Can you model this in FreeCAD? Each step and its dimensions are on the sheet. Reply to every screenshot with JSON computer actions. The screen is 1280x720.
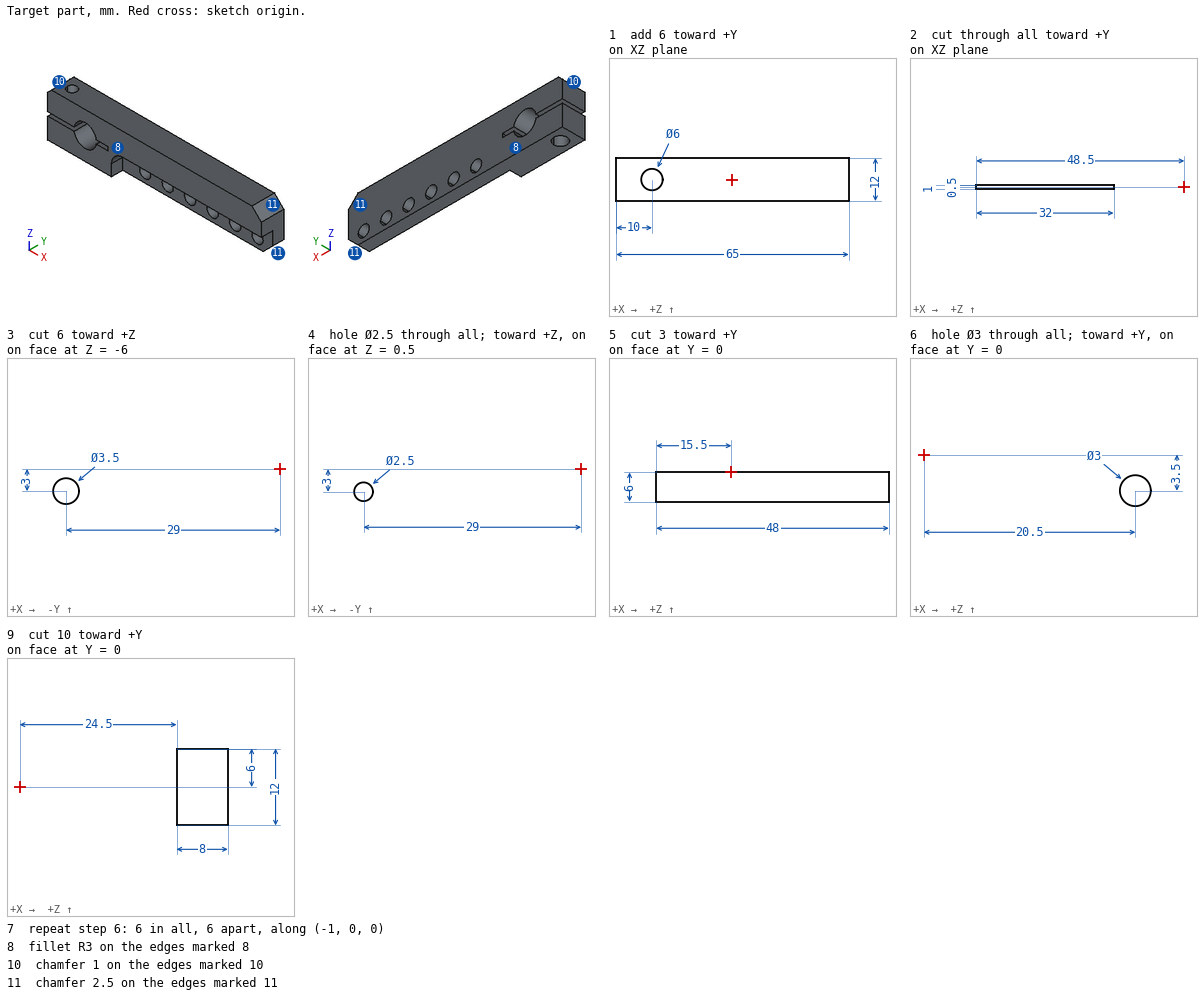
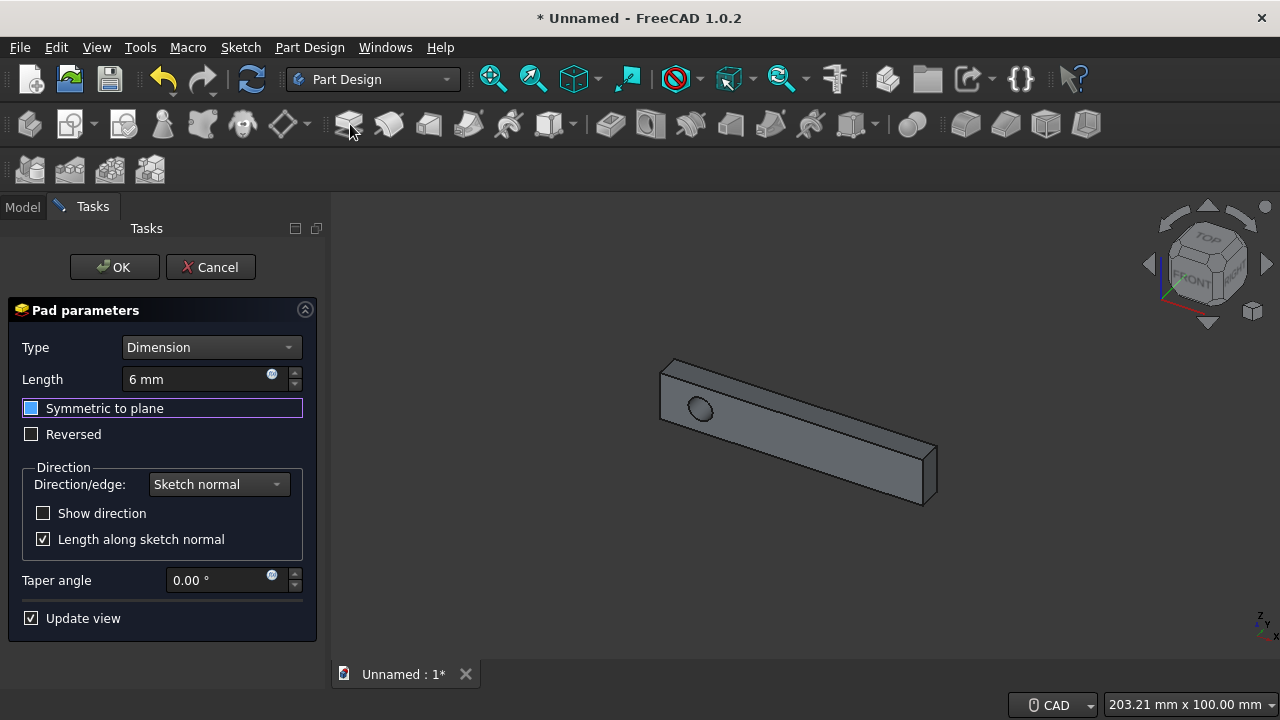
{"action": "left_click", "coordinate": [30, 434]}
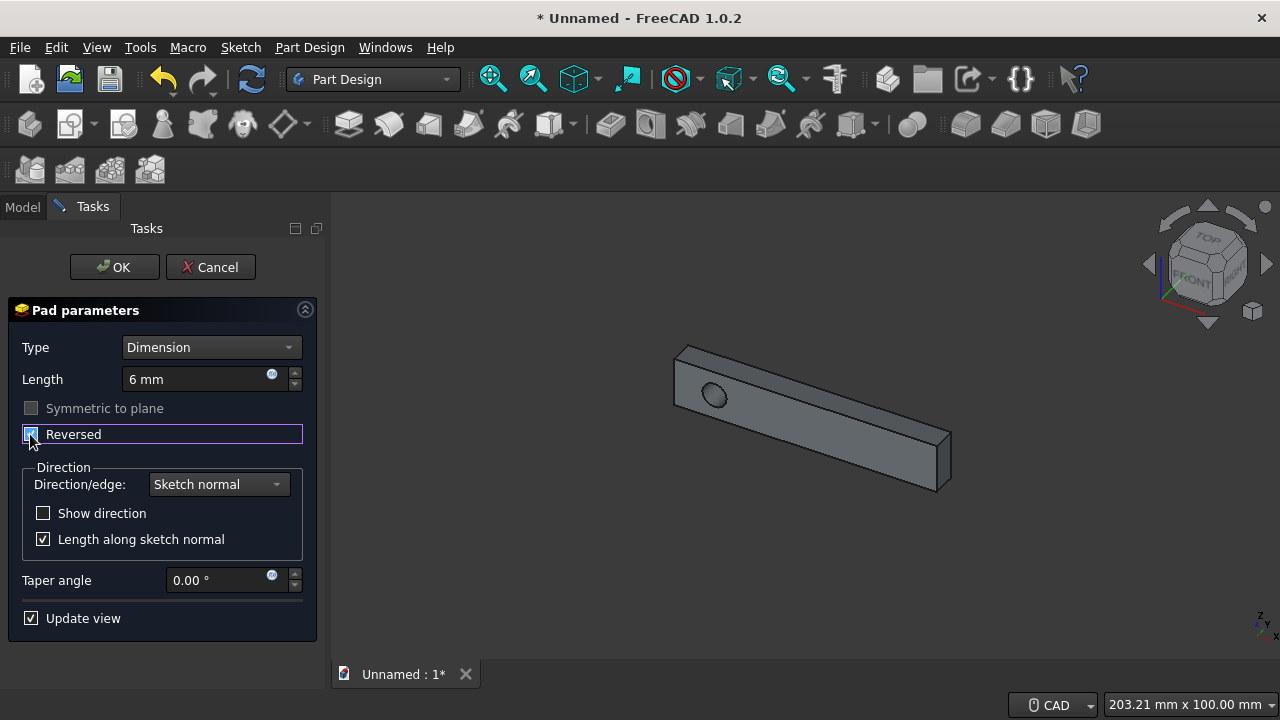
{"action": "left_click", "coordinate": [115, 267]}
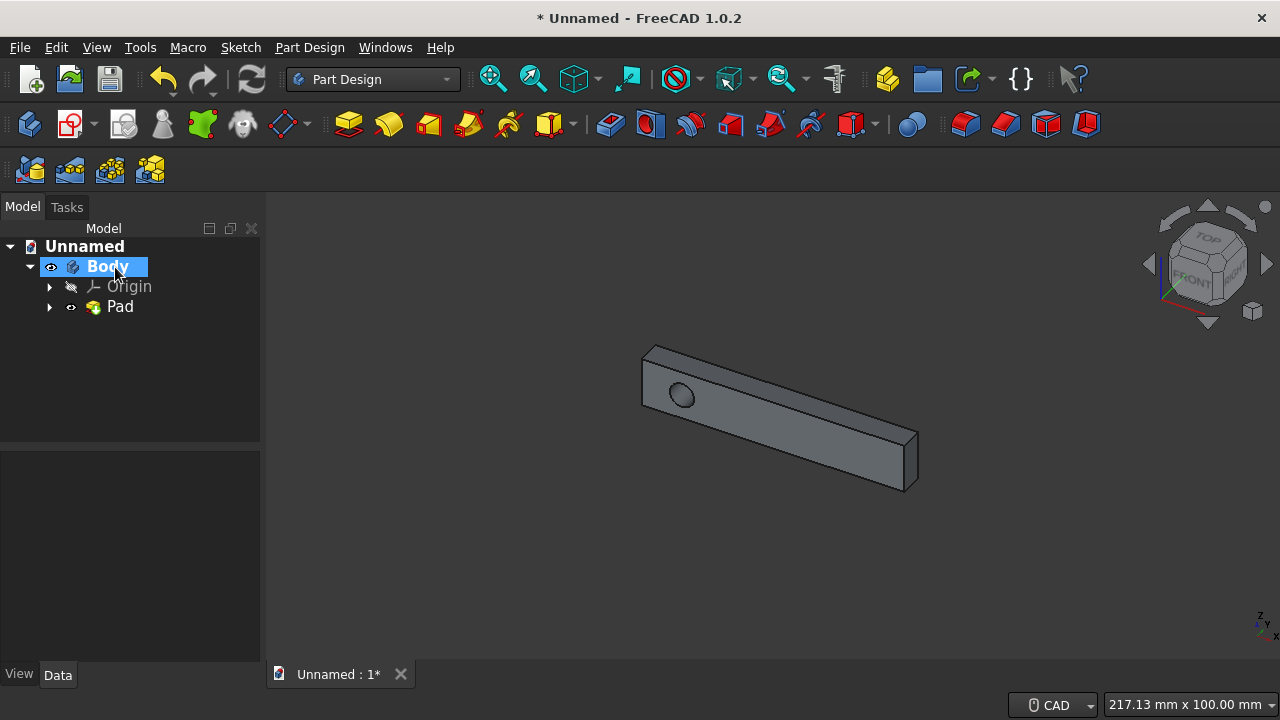
{"action": "left_click", "coordinate": [494, 80]}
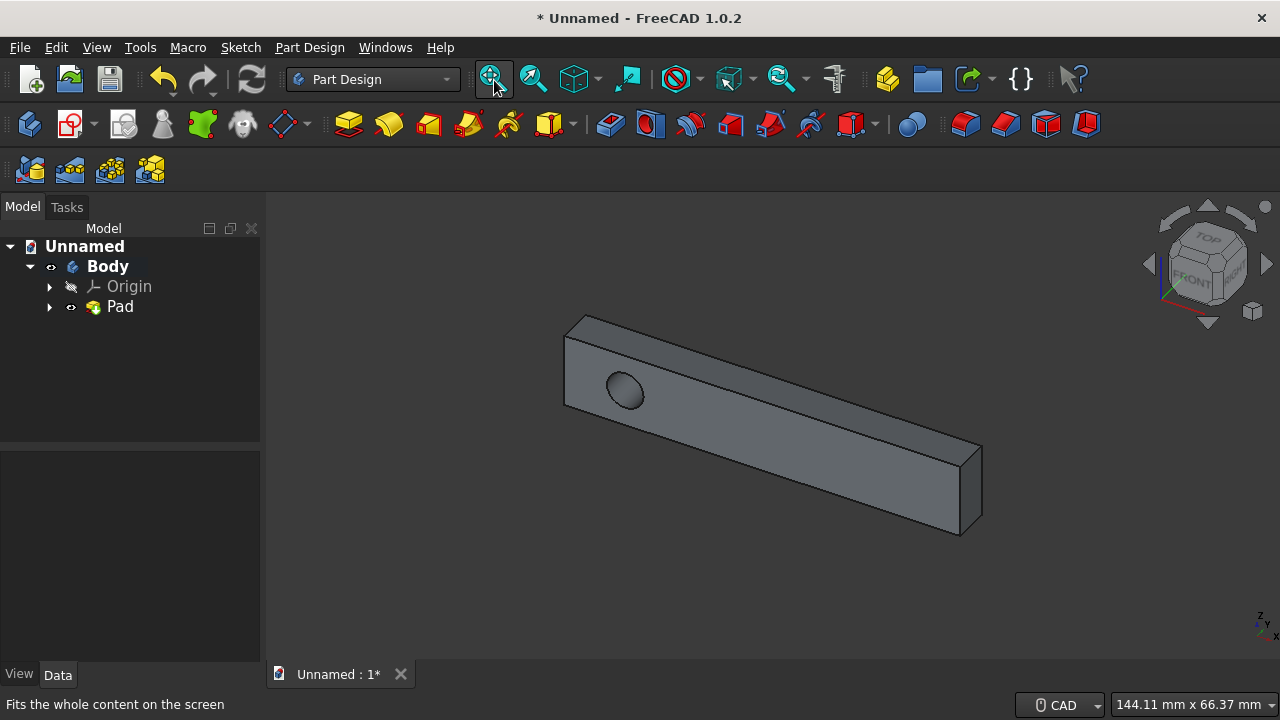
{"action": "left_click", "coordinate": [70, 124]}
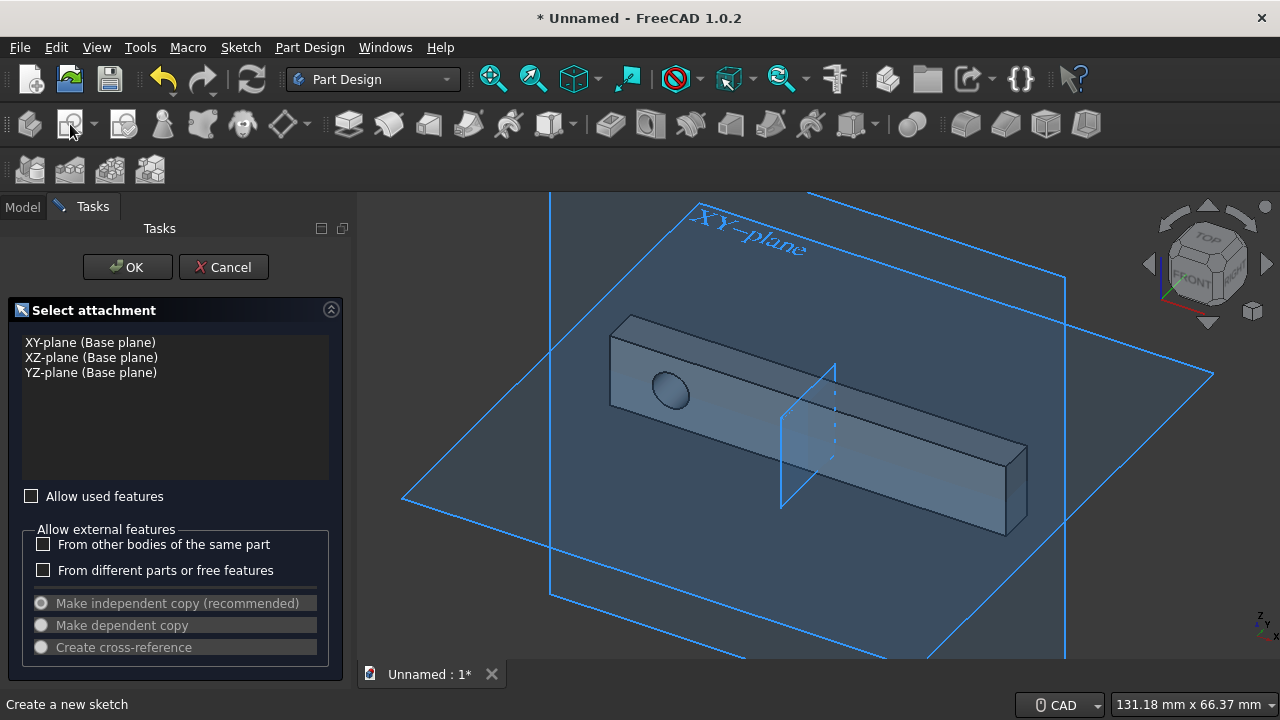
{"action": "left_click", "coordinate": [82, 358]}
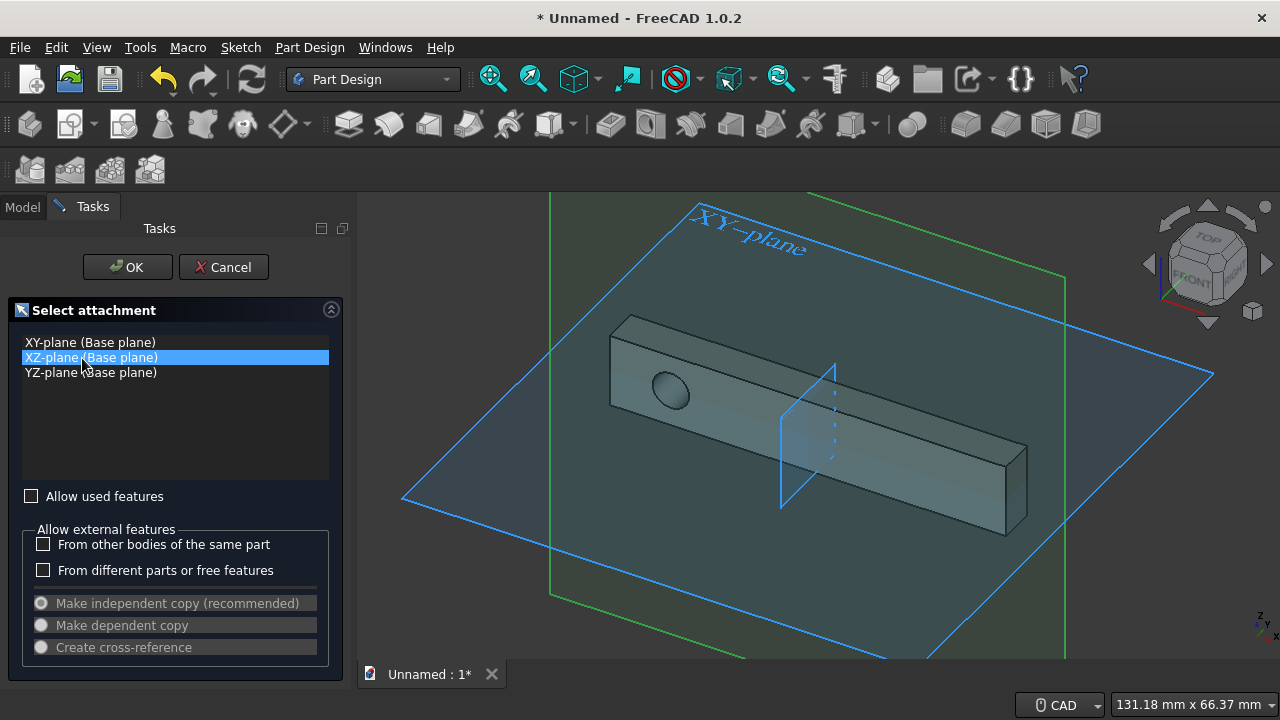
{"action": "left_click", "coordinate": [128, 267]}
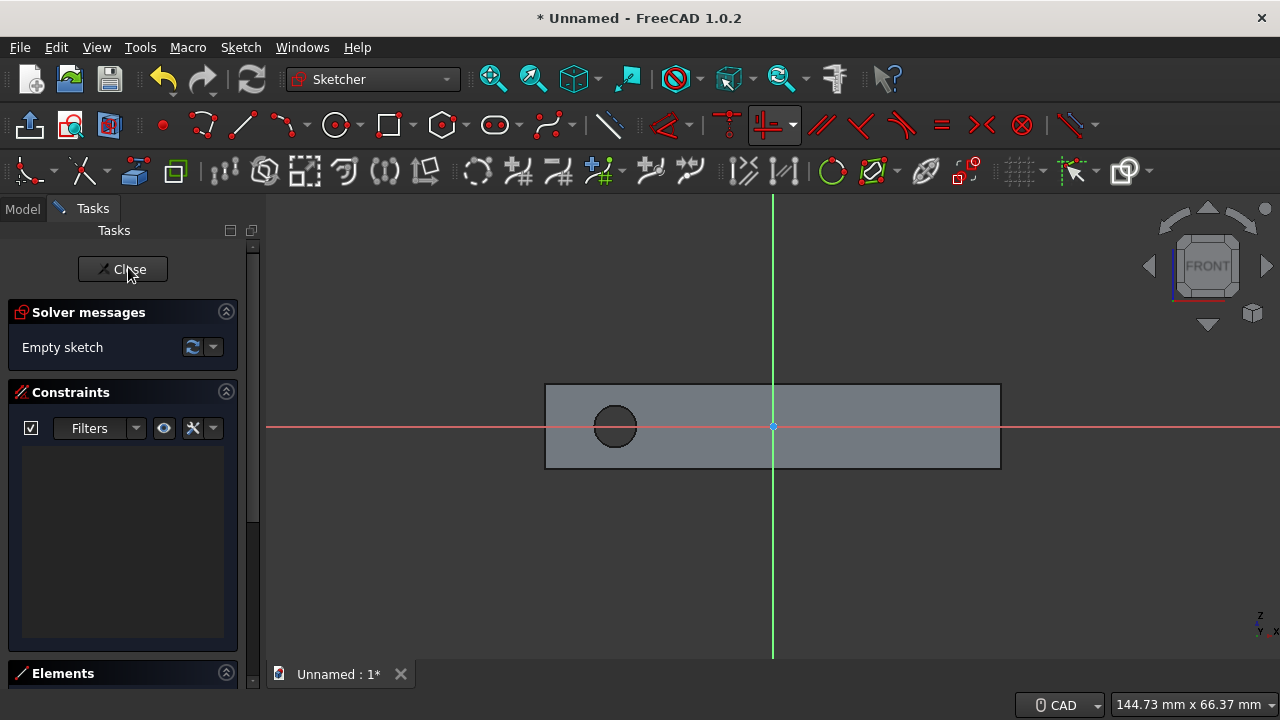
{"action": "scroll", "coordinate": [480, 426], "scroll_direction": "up", "scroll_amount": 3}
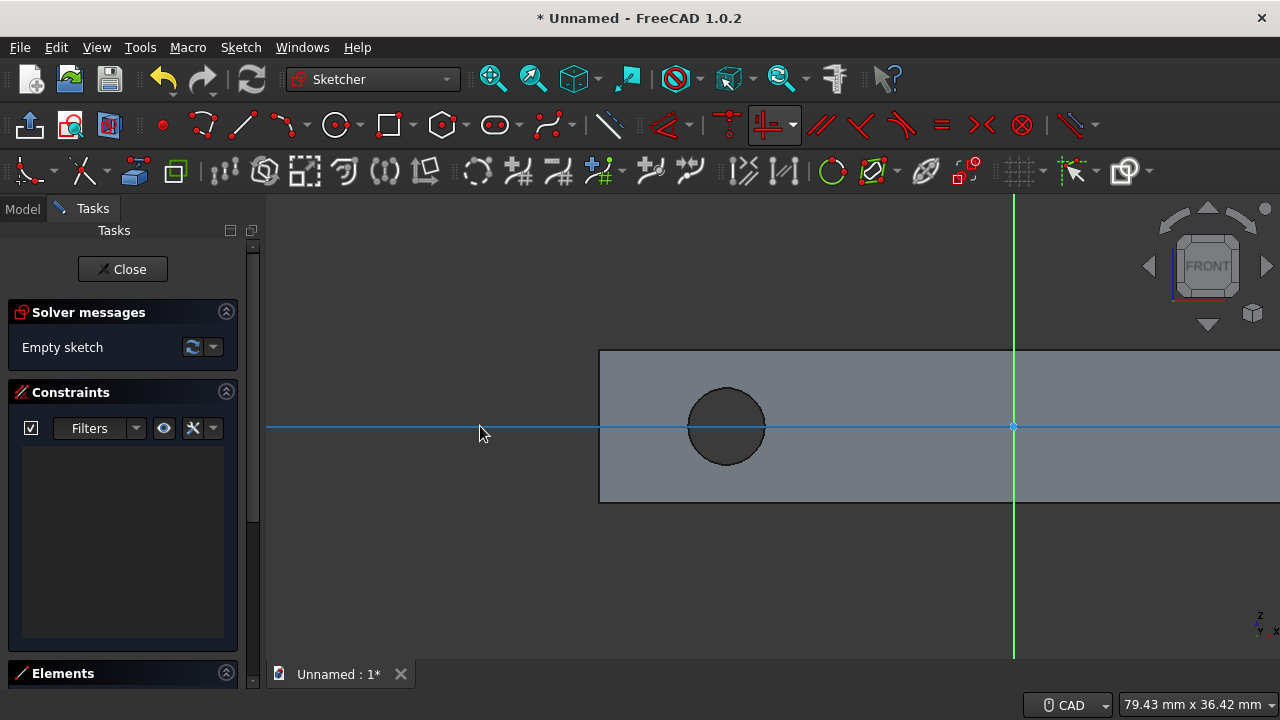
{"action": "left_click", "coordinate": [390, 126]}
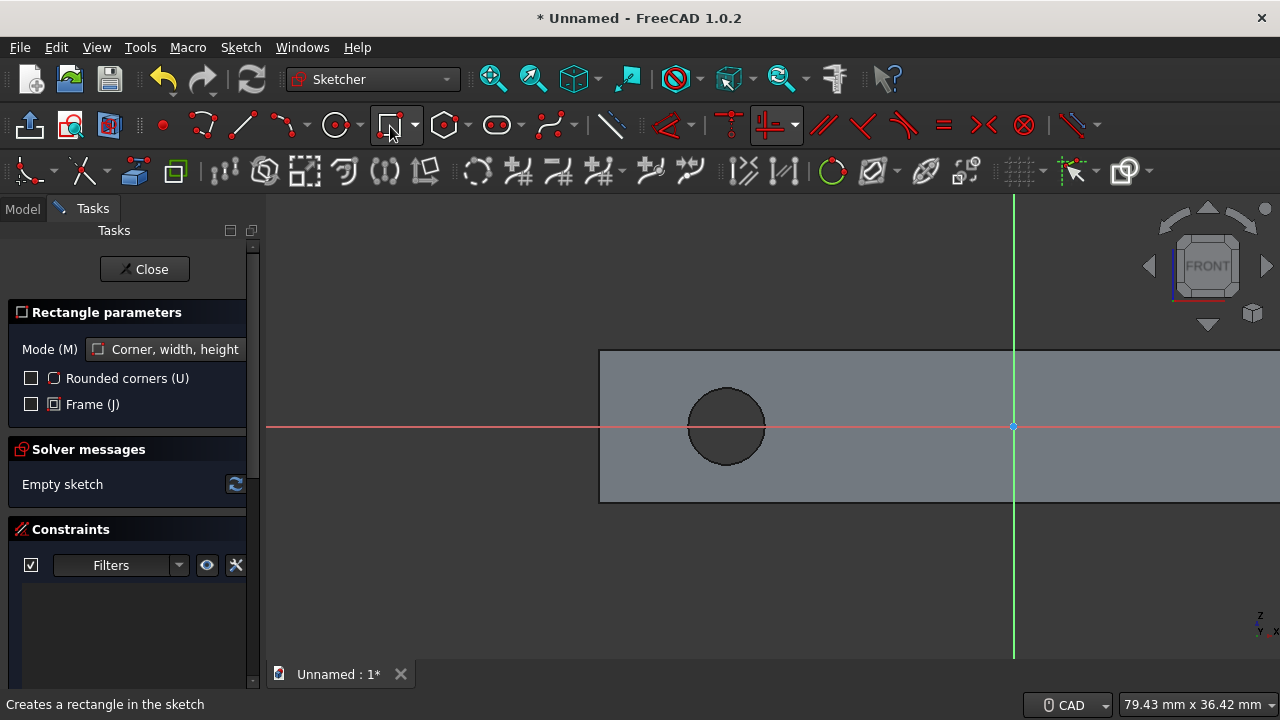
{"action": "scroll", "coordinate": [395, 420], "scroll_direction": "up", "scroll_amount": 5}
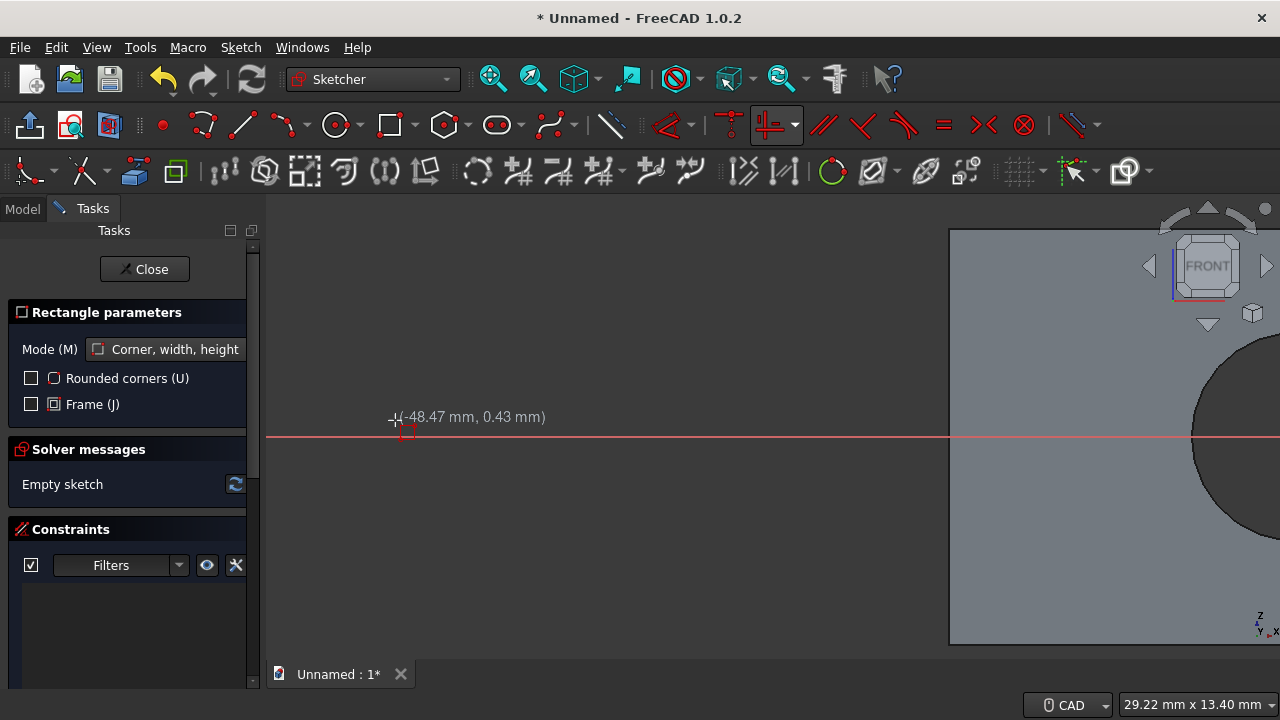
{"action": "left_click", "coordinate": [394, 419]}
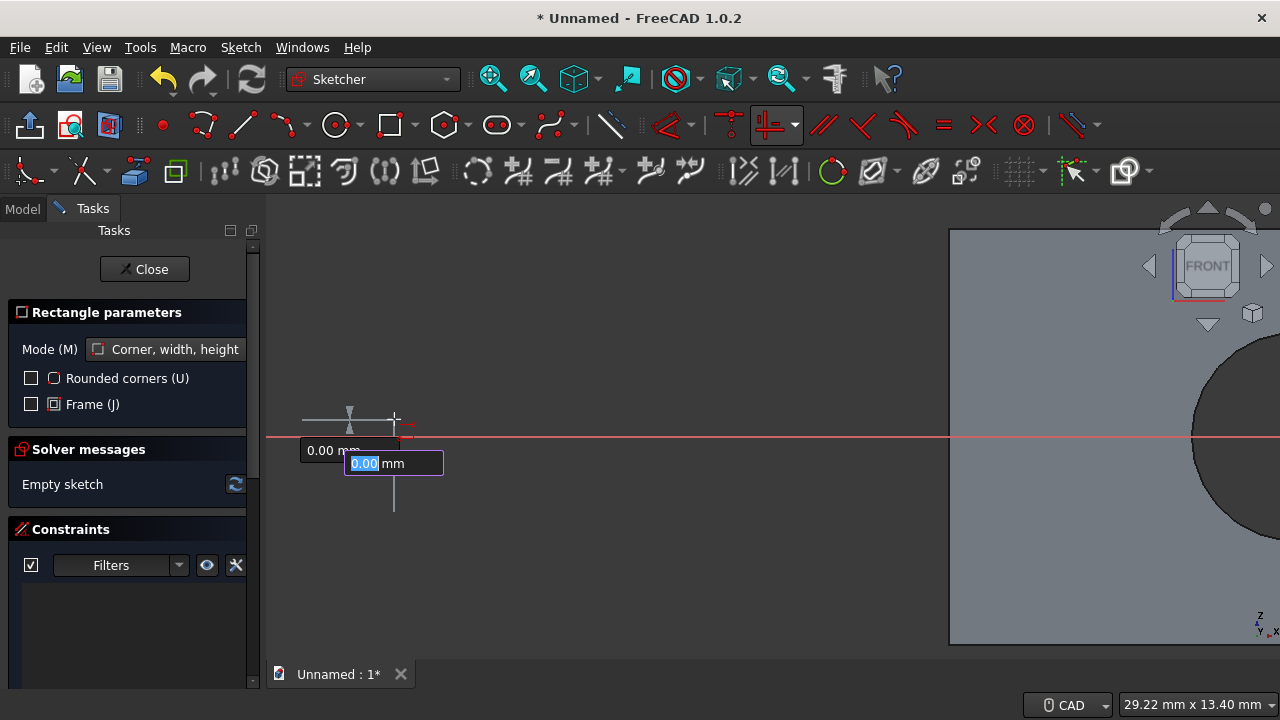
{"action": "scroll", "coordinate": [396, 420], "scroll_direction": "down", "scroll_amount": 5}